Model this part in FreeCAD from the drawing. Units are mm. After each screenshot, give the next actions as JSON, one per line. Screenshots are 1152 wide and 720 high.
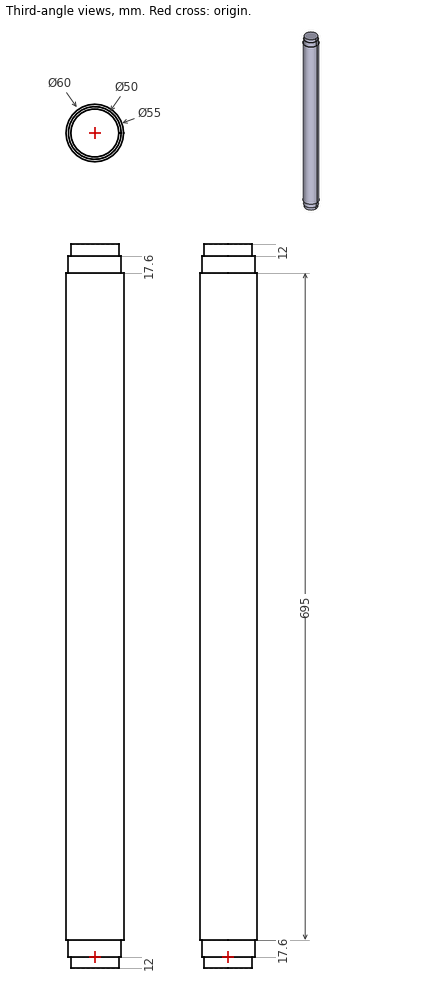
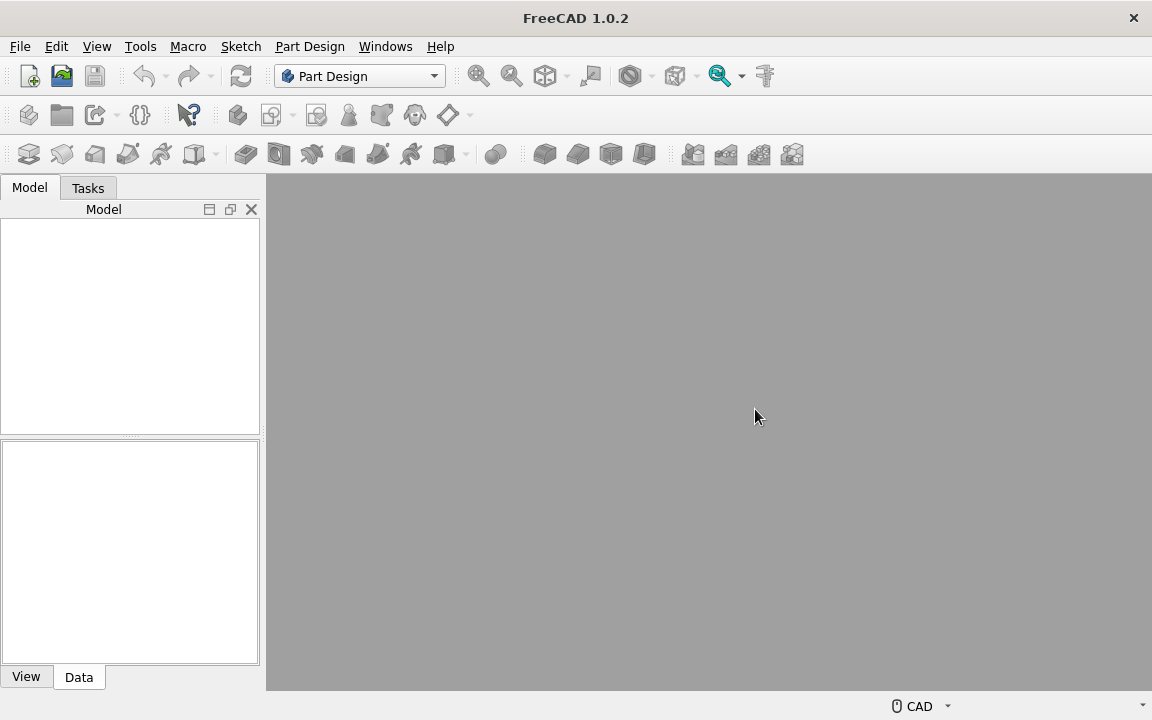
{"action": "left_click", "coordinate": [29, 76]}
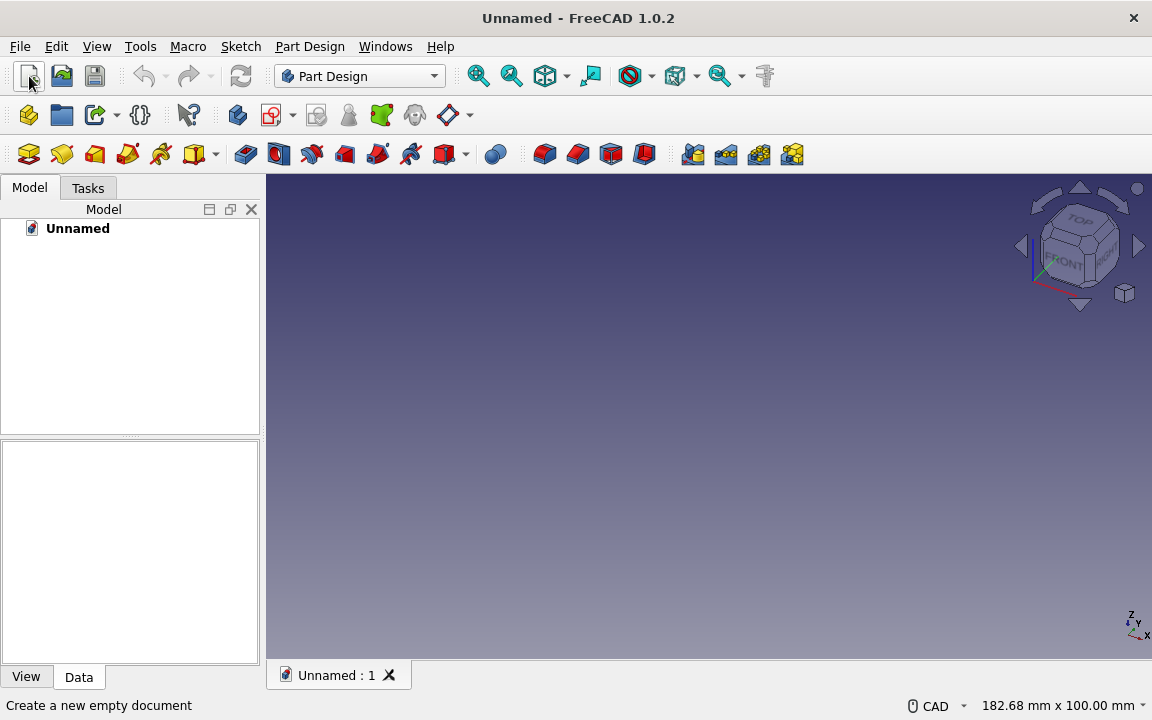
{"action": "left_click", "coordinate": [270, 116]}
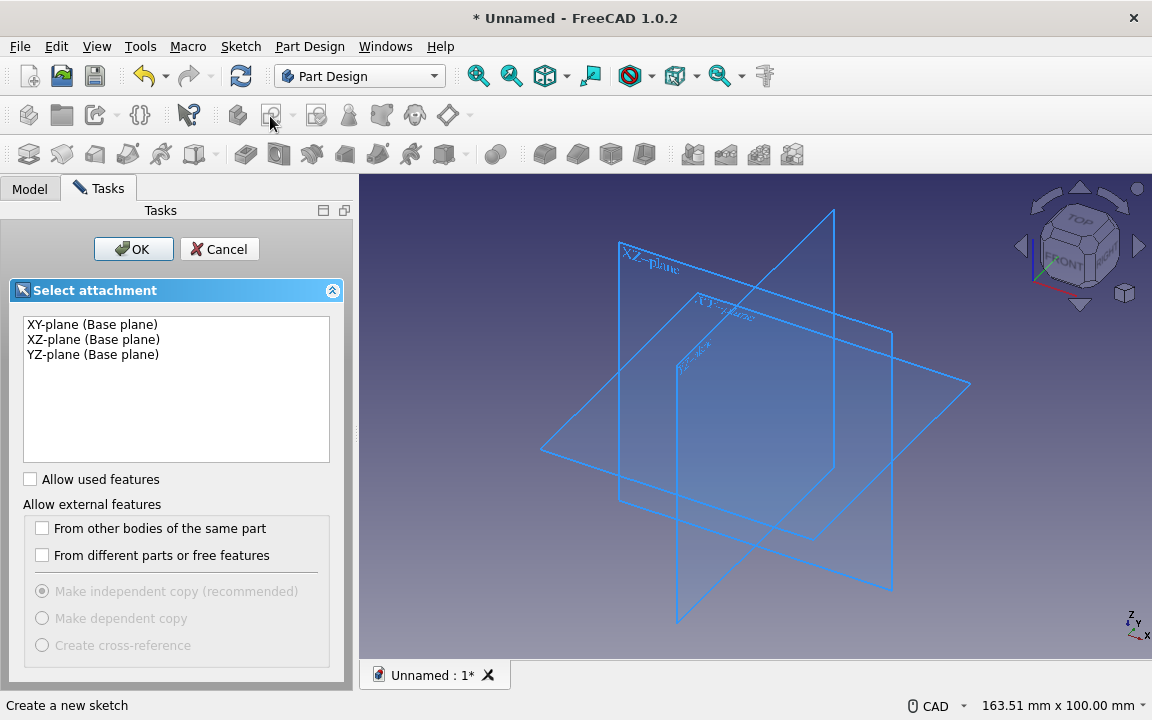
{"action": "left_click", "coordinate": [84, 324]}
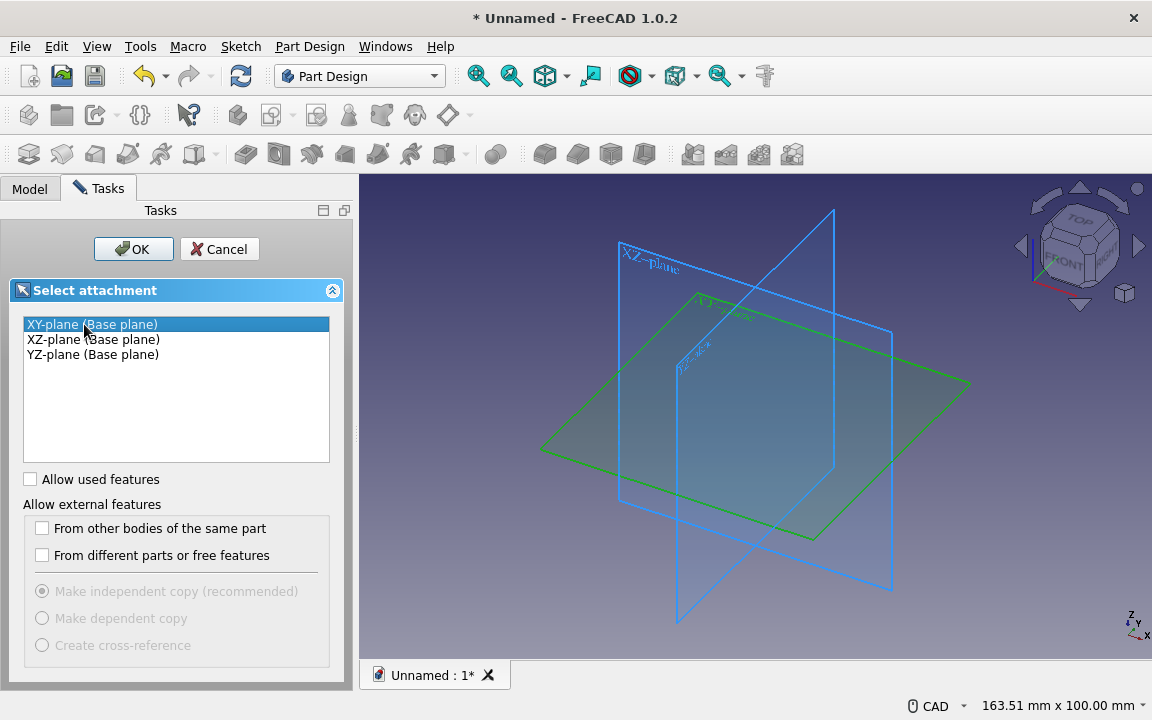
{"action": "left_click", "coordinate": [134, 249]}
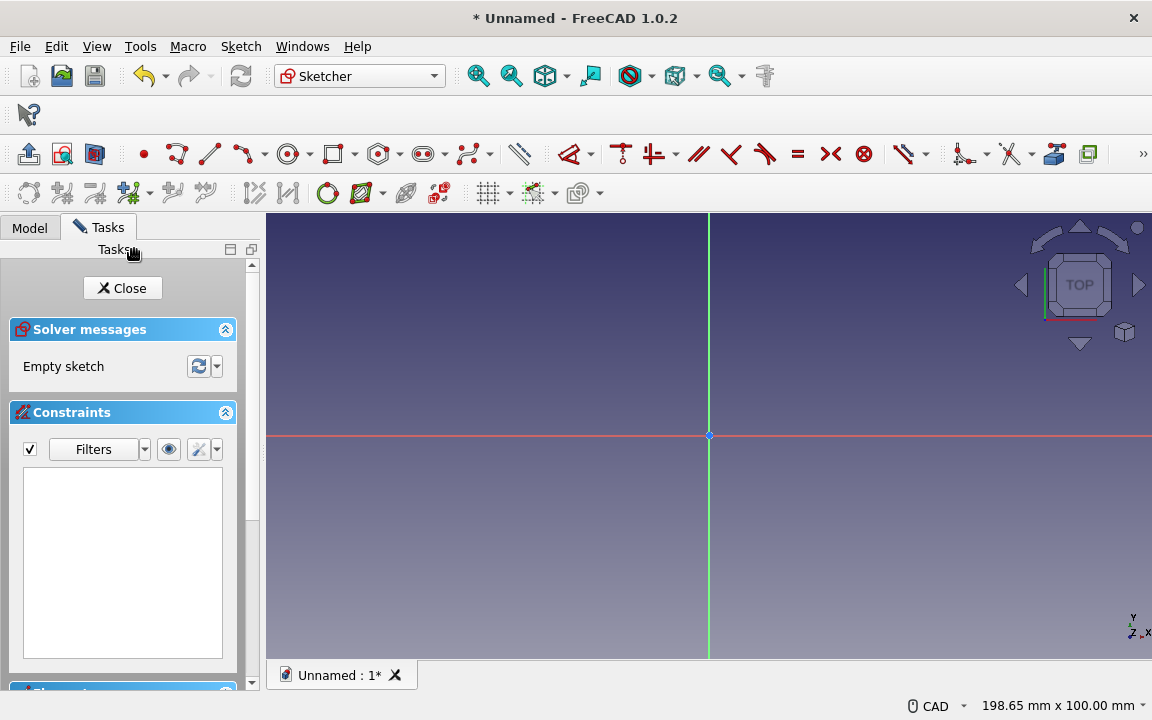
{"action": "left_click", "coordinate": [288, 154]}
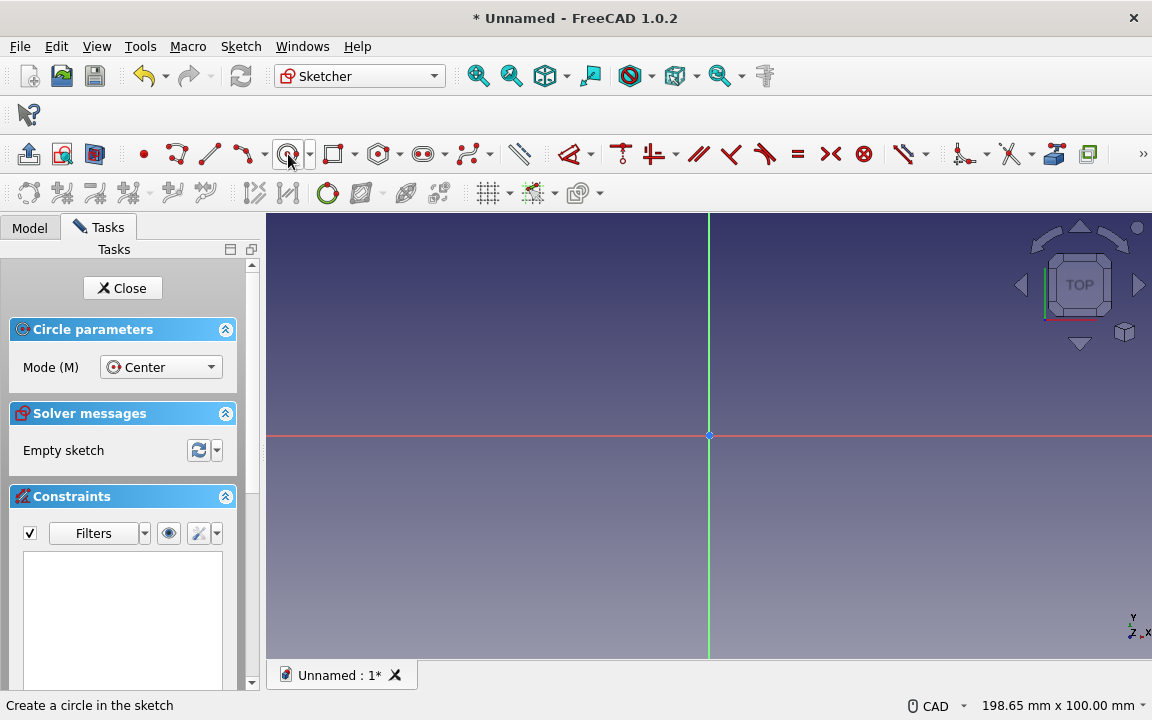
{"action": "left_click", "coordinate": [709, 436]}
{"action": "mouse_move", "coordinate": [796, 349]}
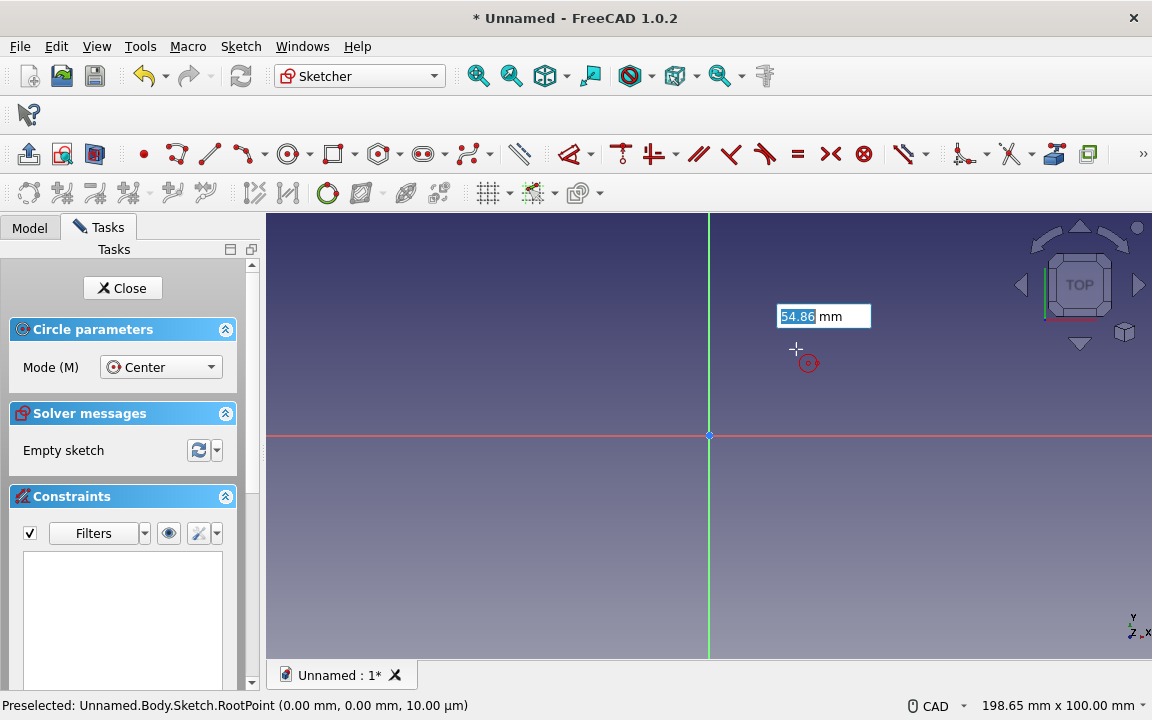
{"action": "type", "text": "55"}
{"action": "key", "text": "Return"}
{"action": "key", "text": "Escape"}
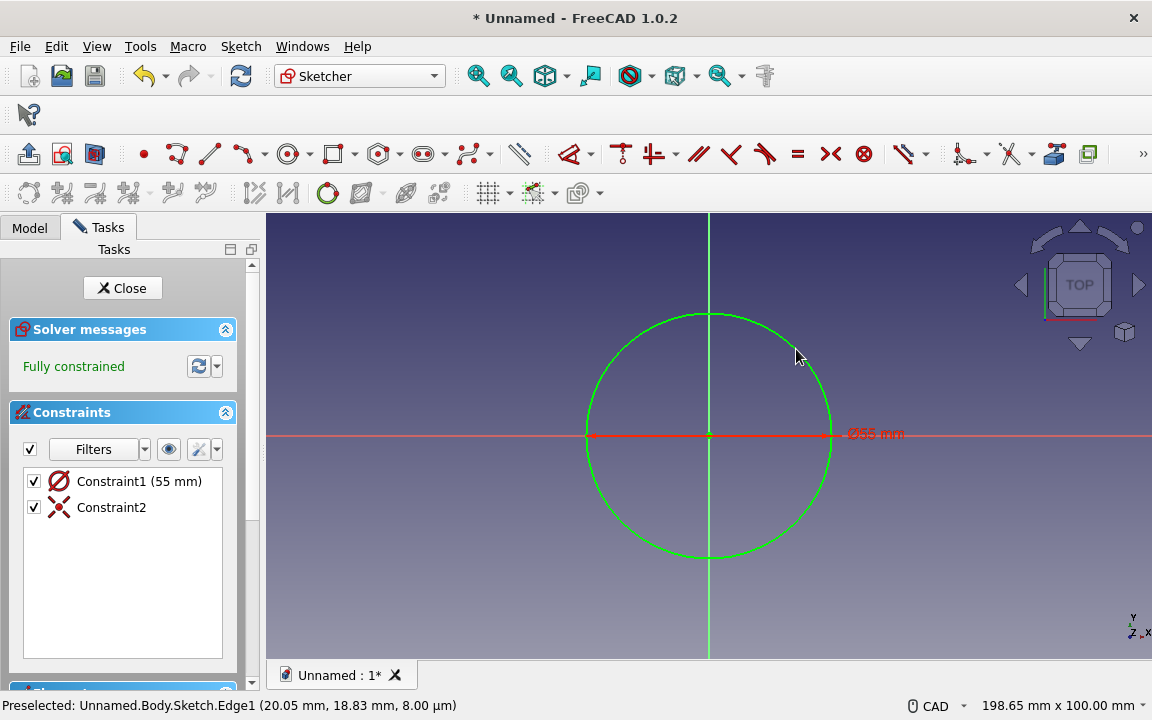
{"action": "left_click", "coordinate": [123, 288]}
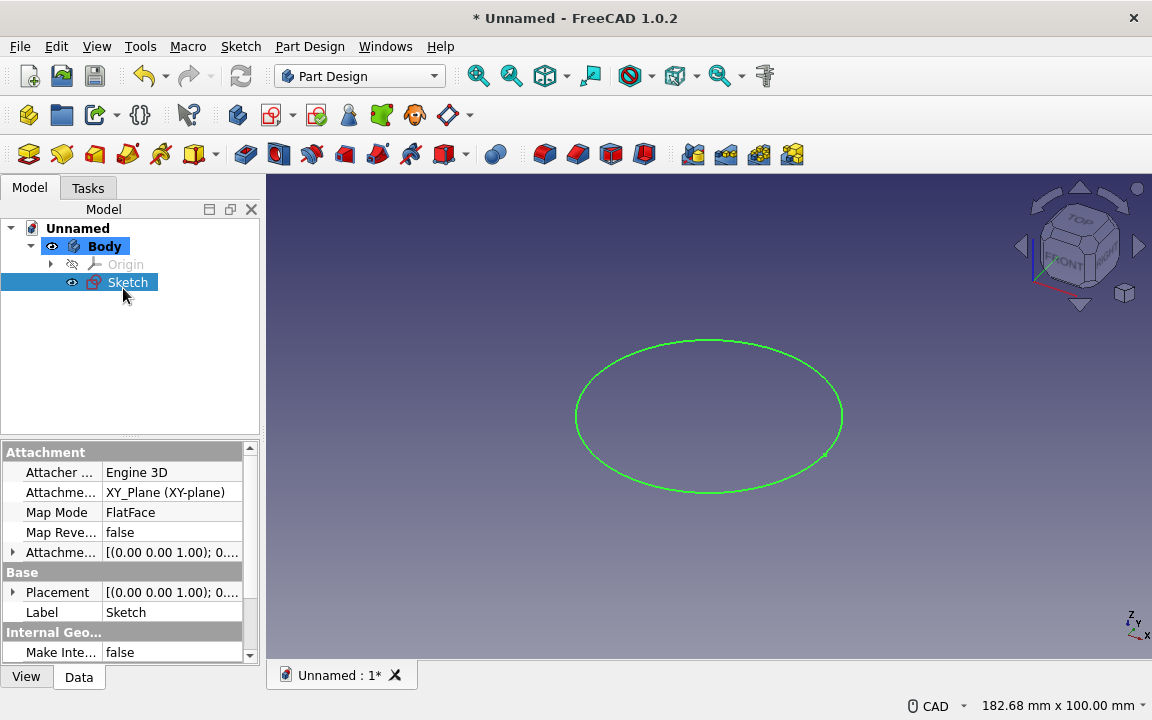
{"action": "left_click", "coordinate": [29, 154]}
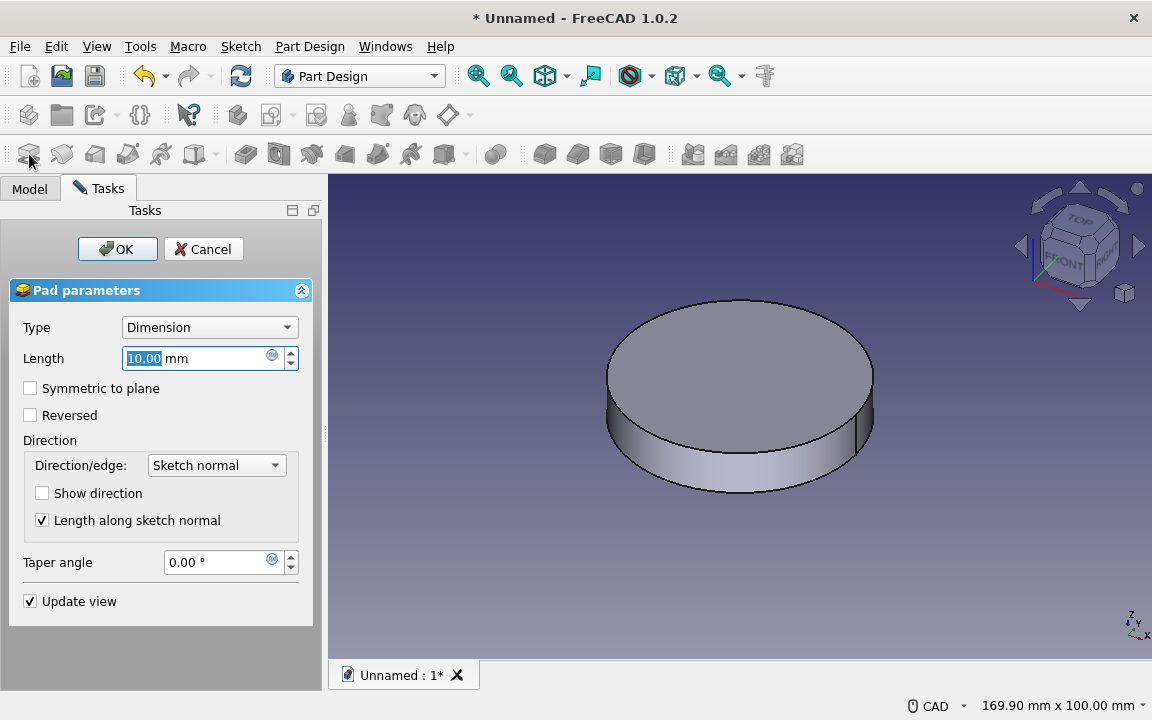
{"action": "type", "text": "17.6"}
{"action": "key", "text": "Tab"}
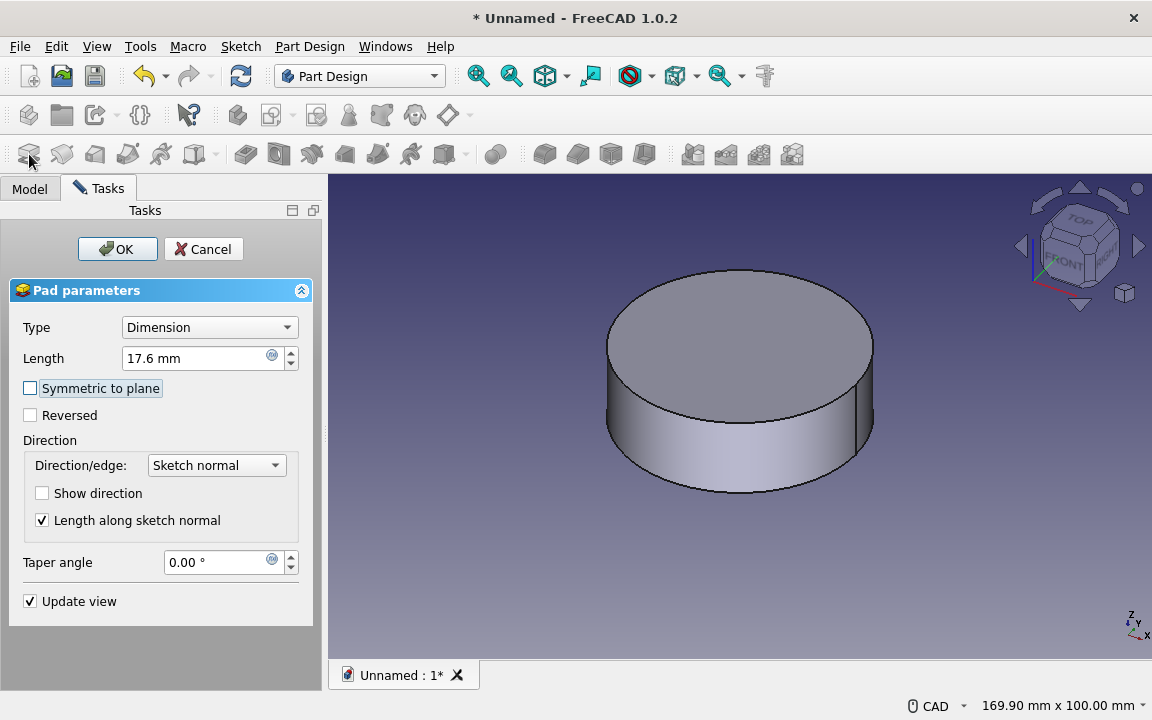
{"action": "left_click", "coordinate": [118, 249]}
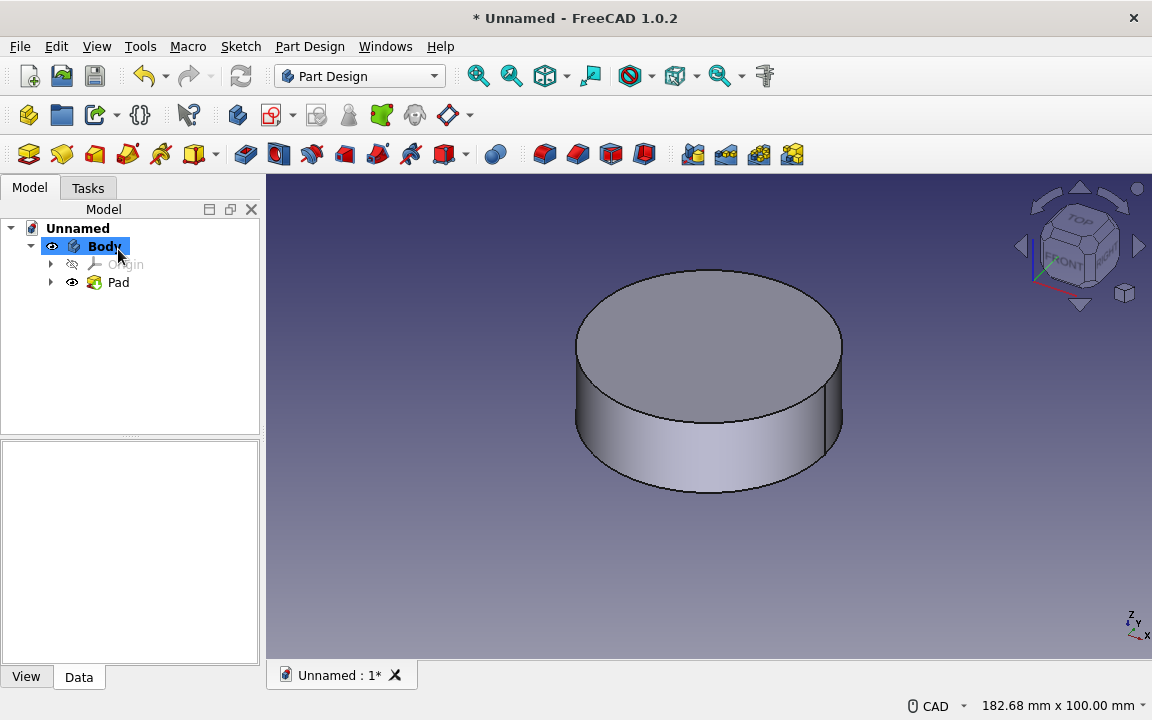
{"action": "left_click", "coordinate": [270, 116]}